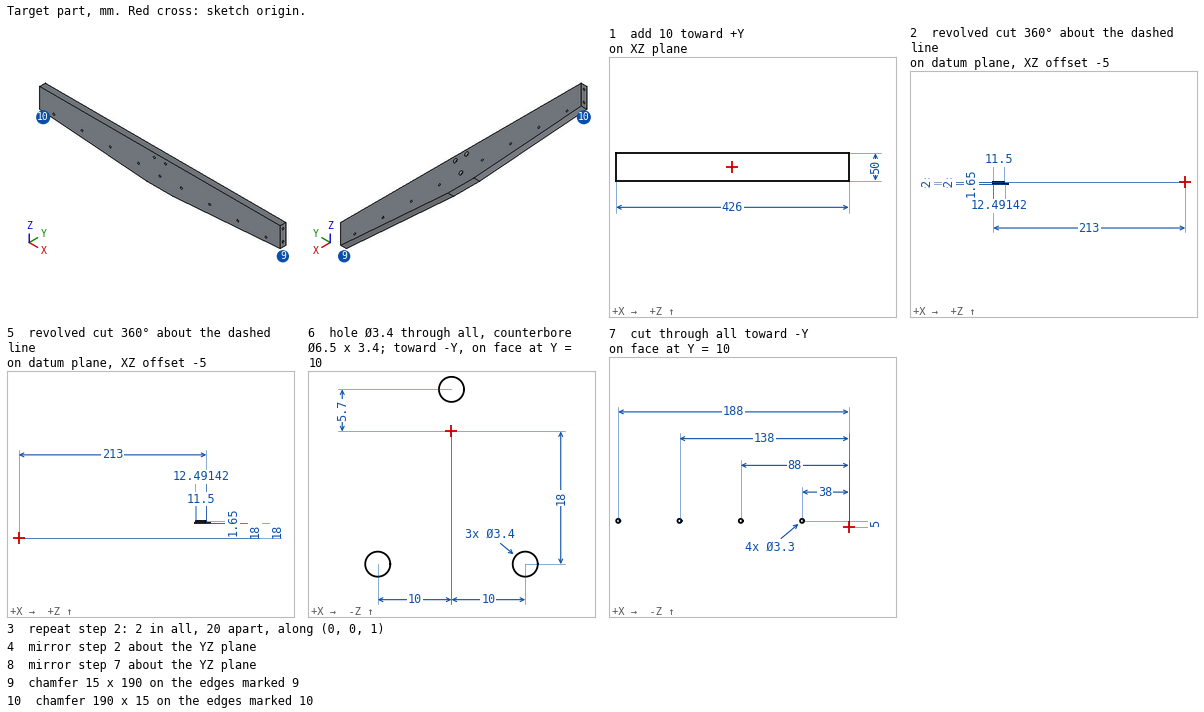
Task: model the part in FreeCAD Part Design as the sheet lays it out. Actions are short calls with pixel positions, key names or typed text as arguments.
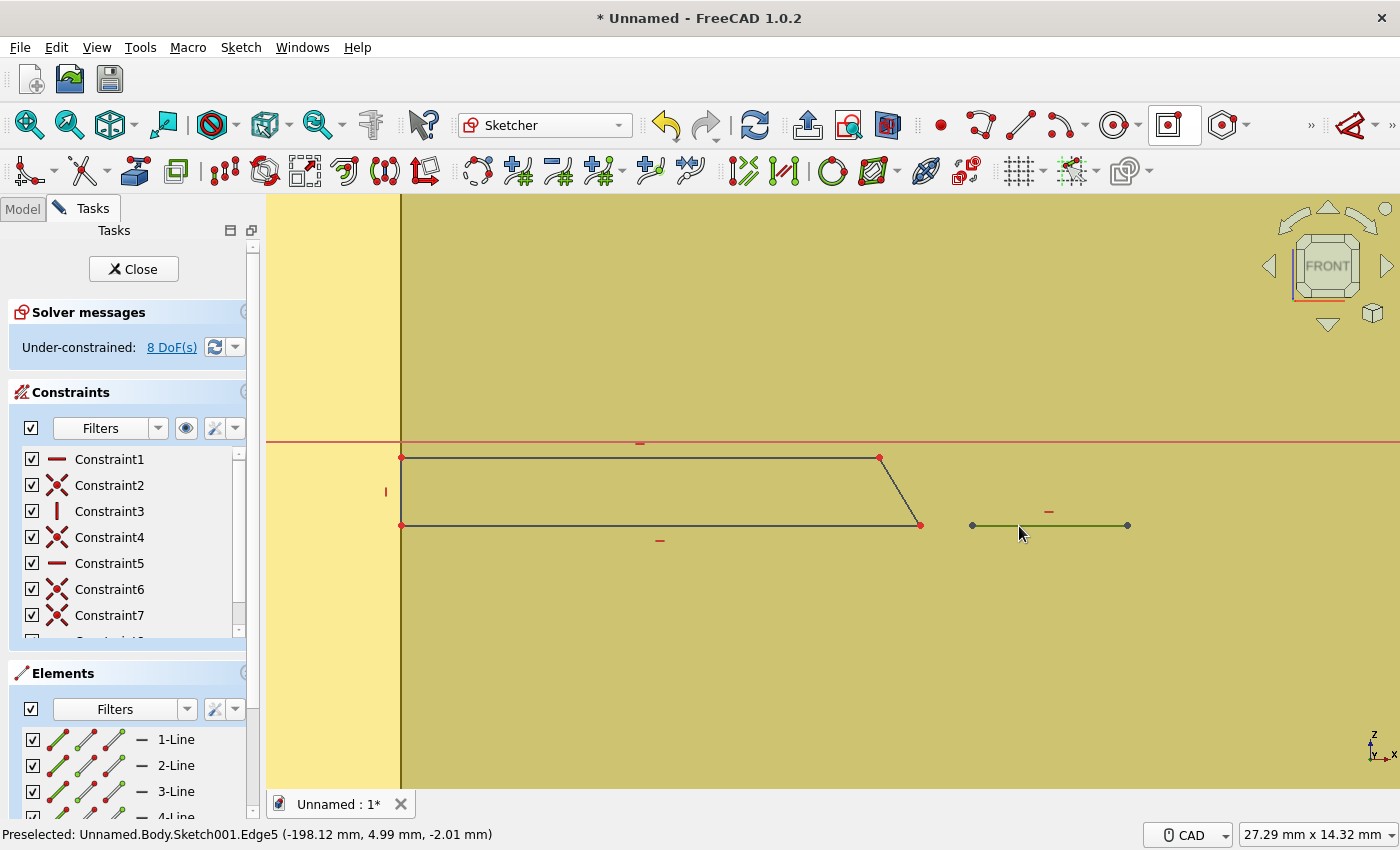
key(g)
key(n)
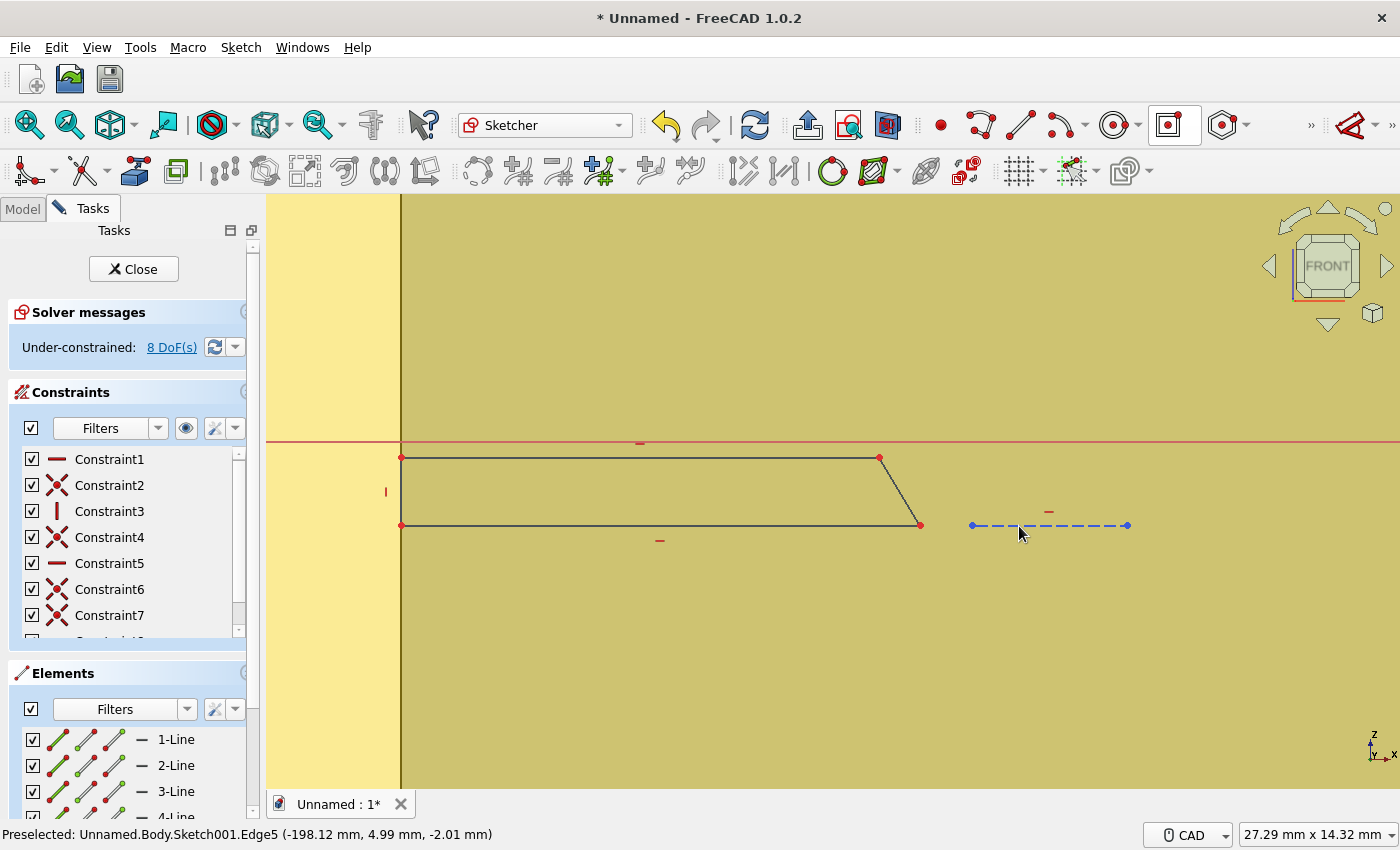
click(1350, 126)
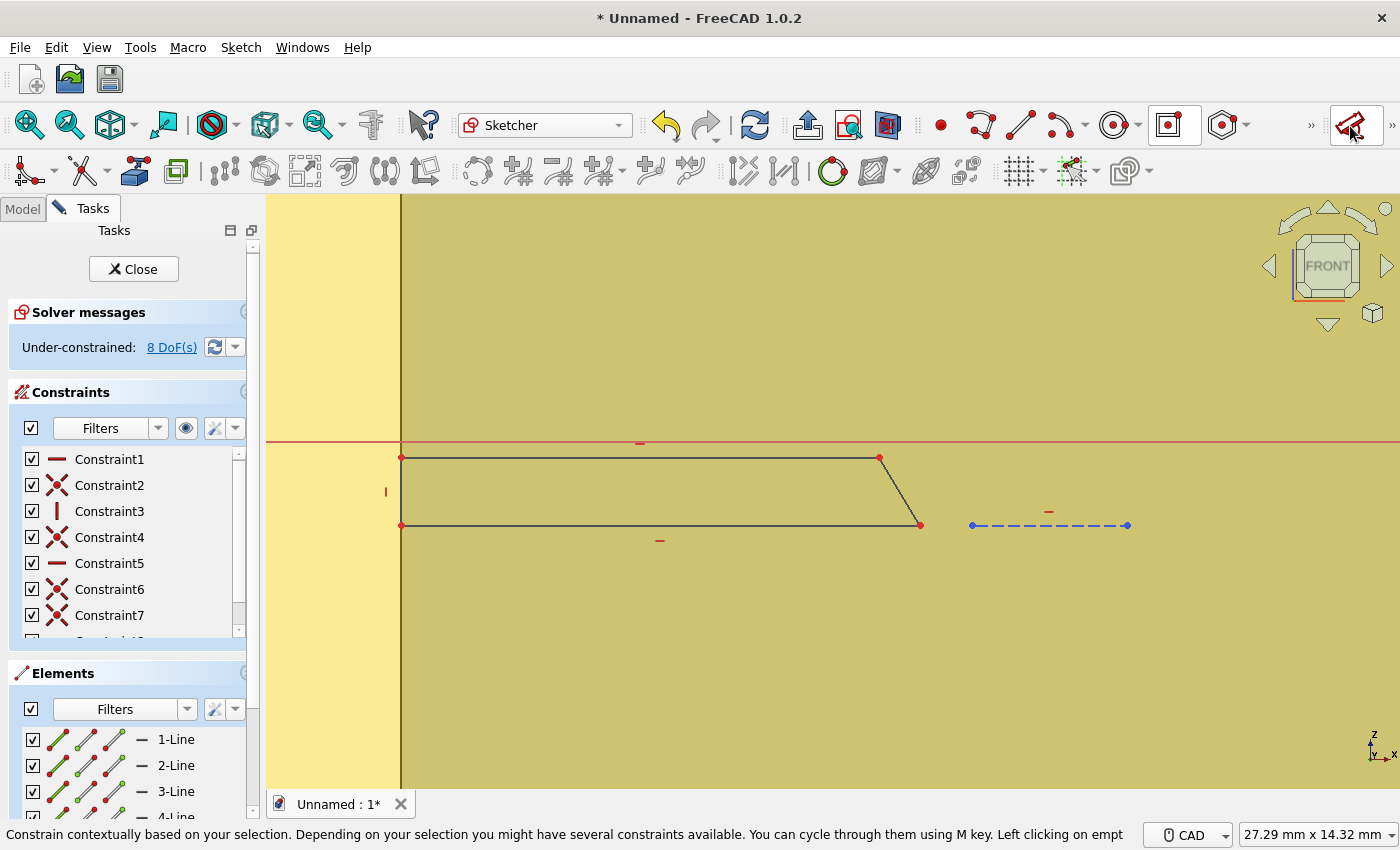
click(920, 526)
click(886, 503)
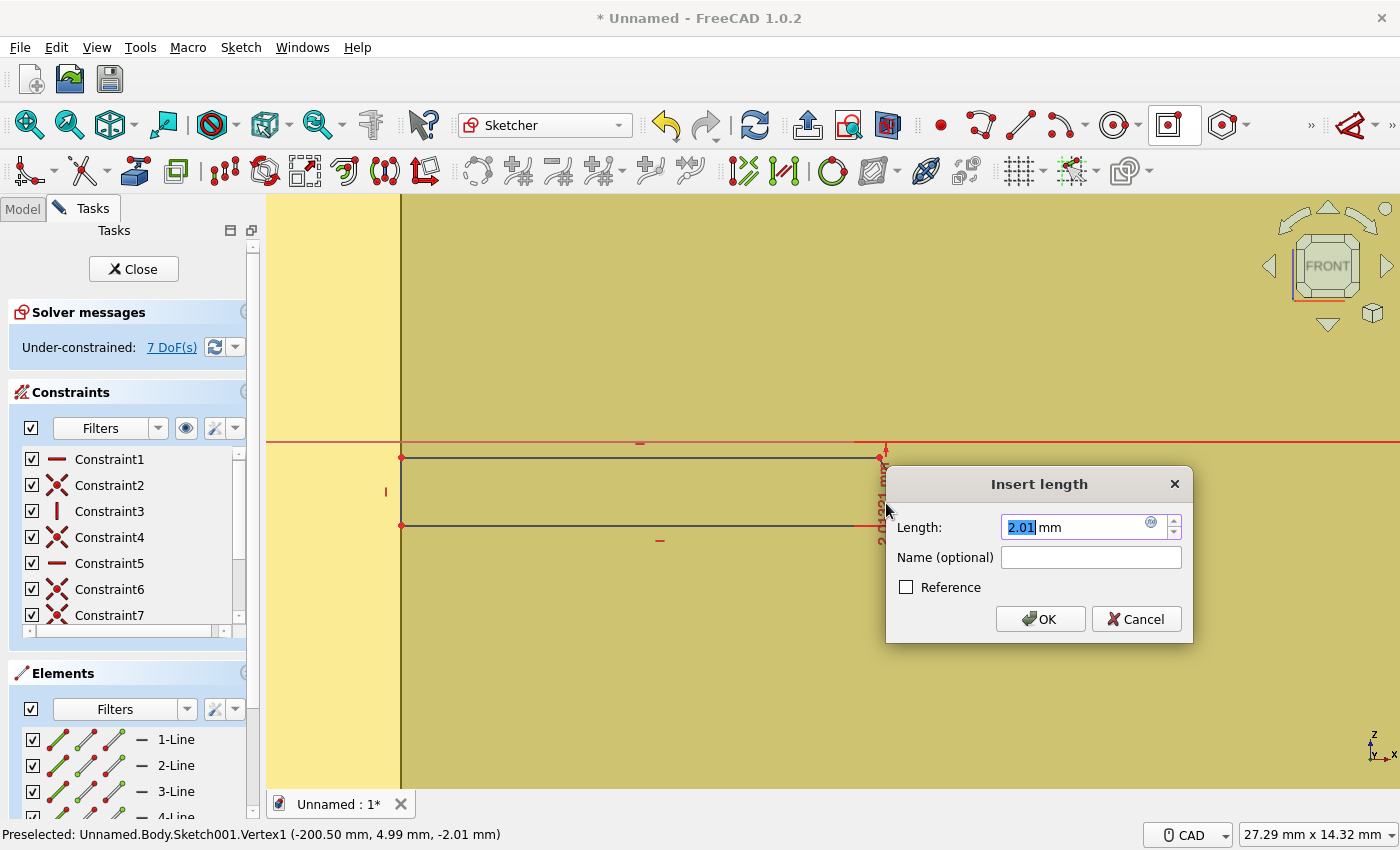
text(2)
key(Return)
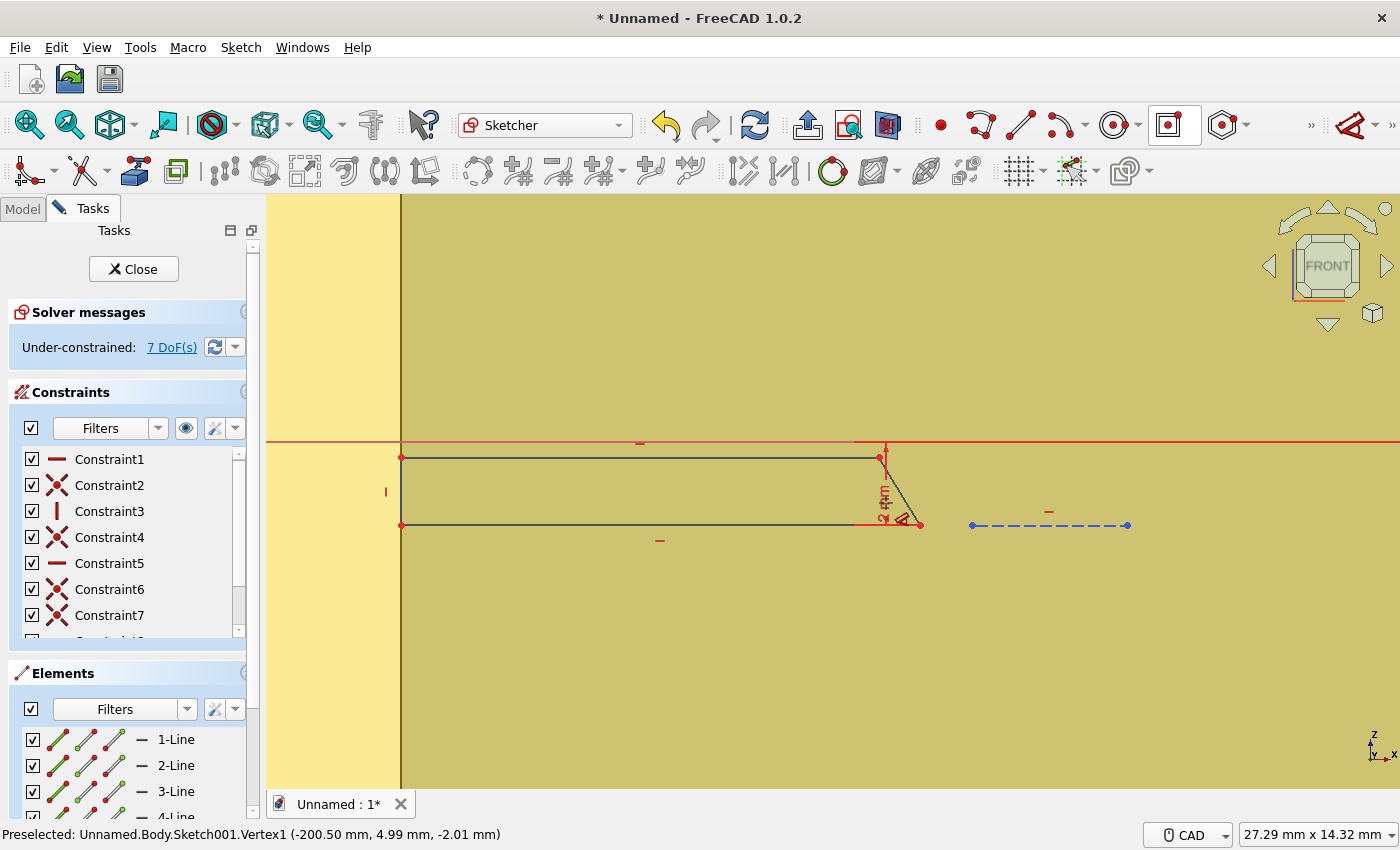
click(972, 526)
click(938, 465)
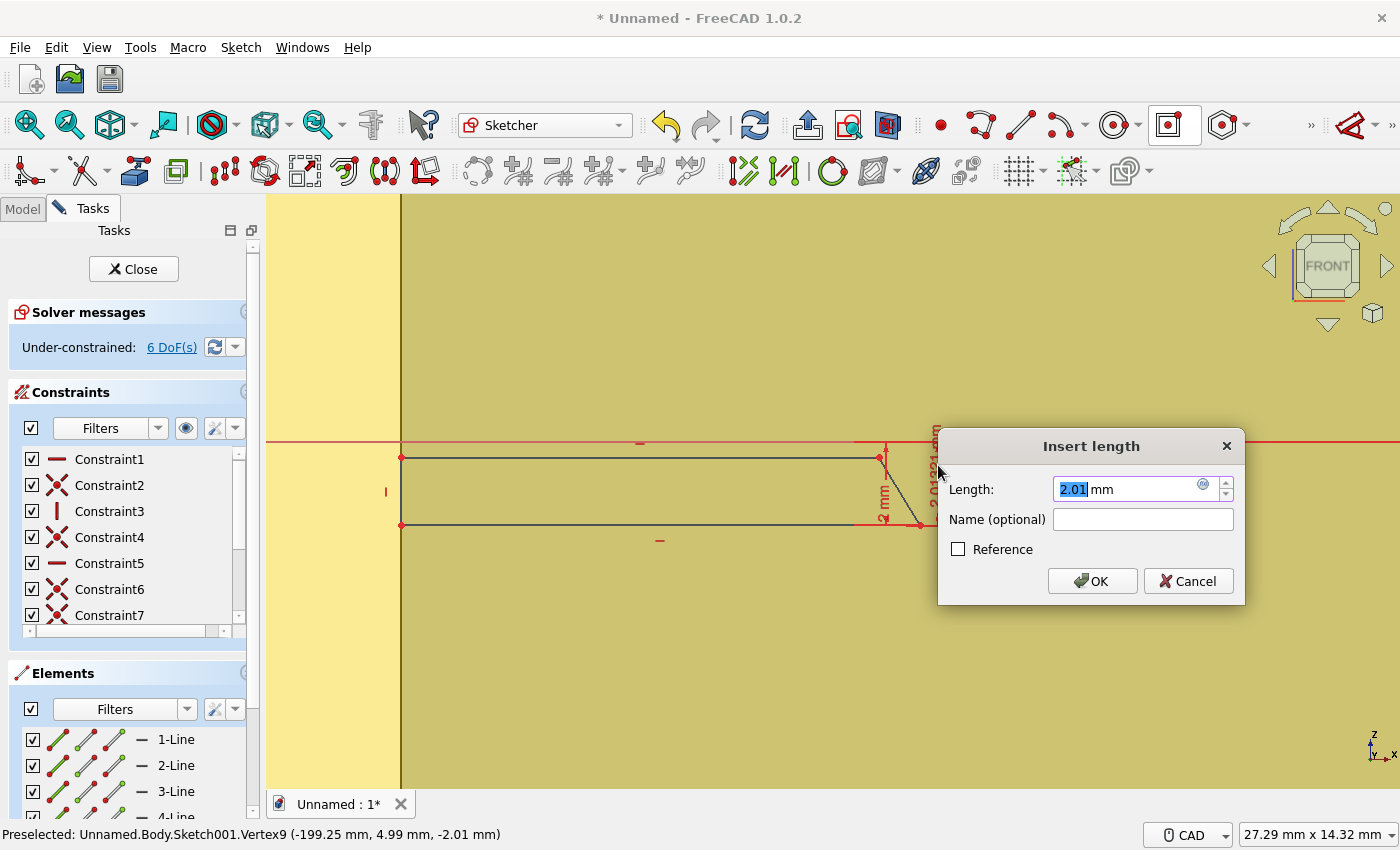
text(2)
key(Return)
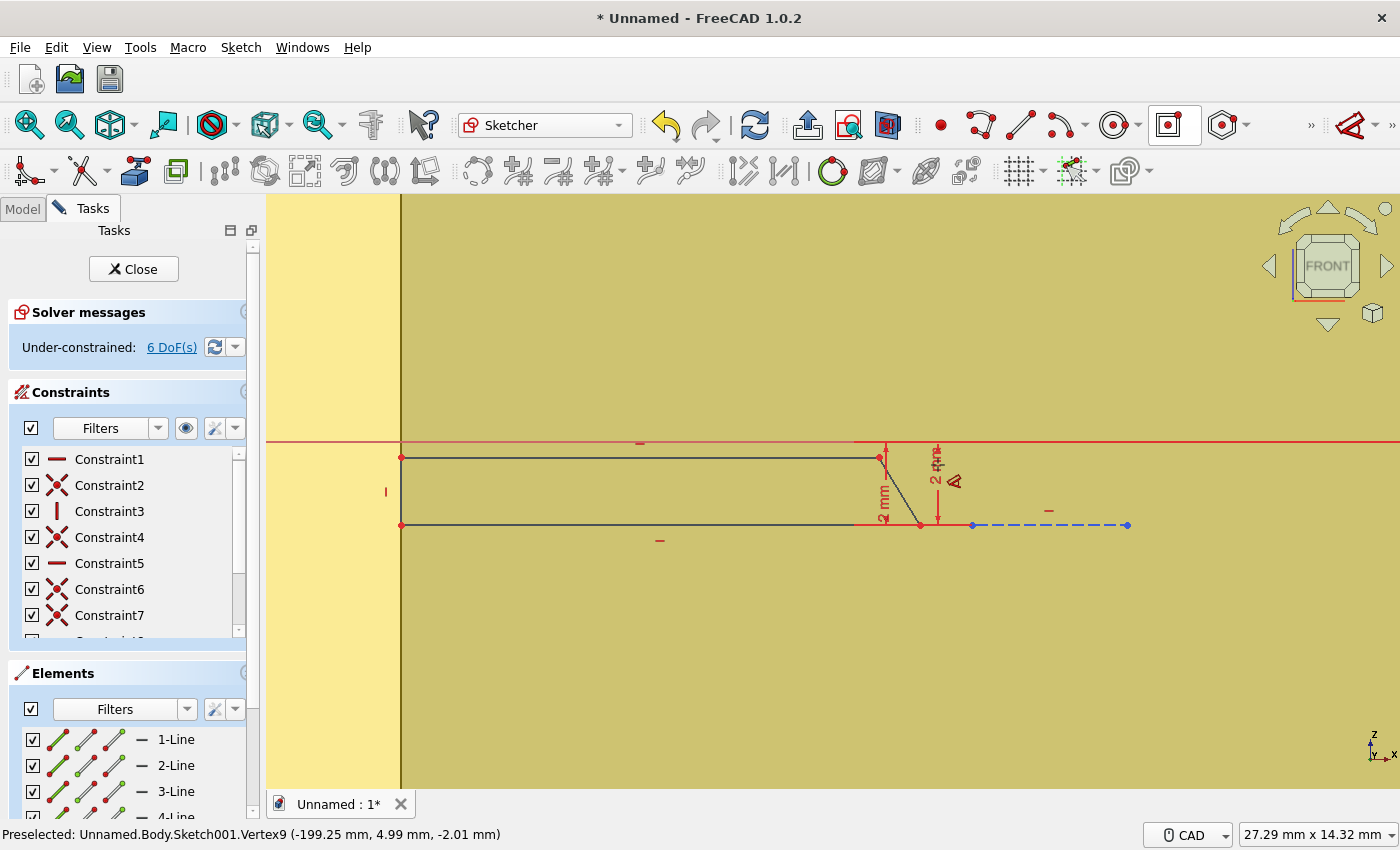
click(401, 505)
click(367, 492)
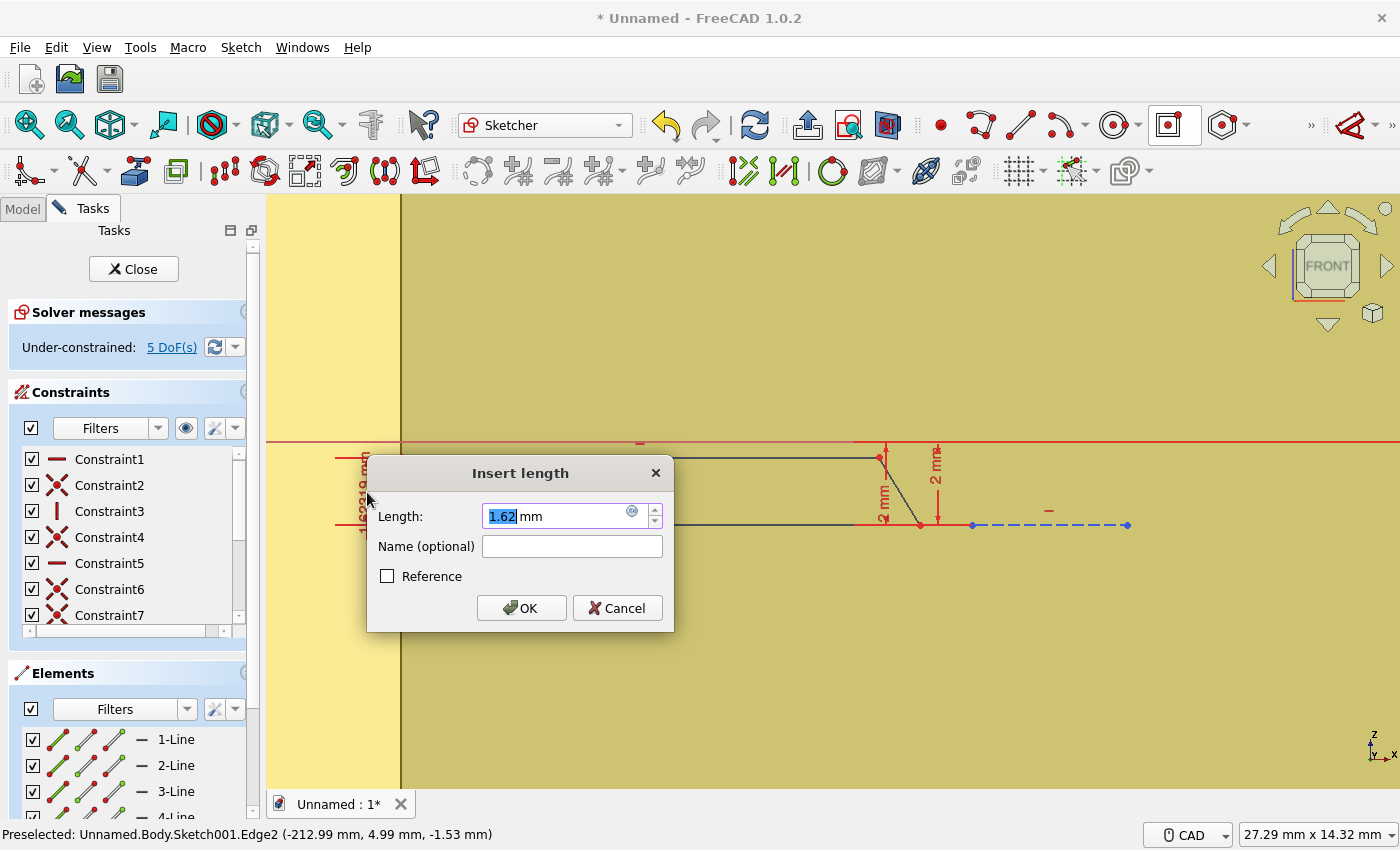
text(1.65)
key(Return)